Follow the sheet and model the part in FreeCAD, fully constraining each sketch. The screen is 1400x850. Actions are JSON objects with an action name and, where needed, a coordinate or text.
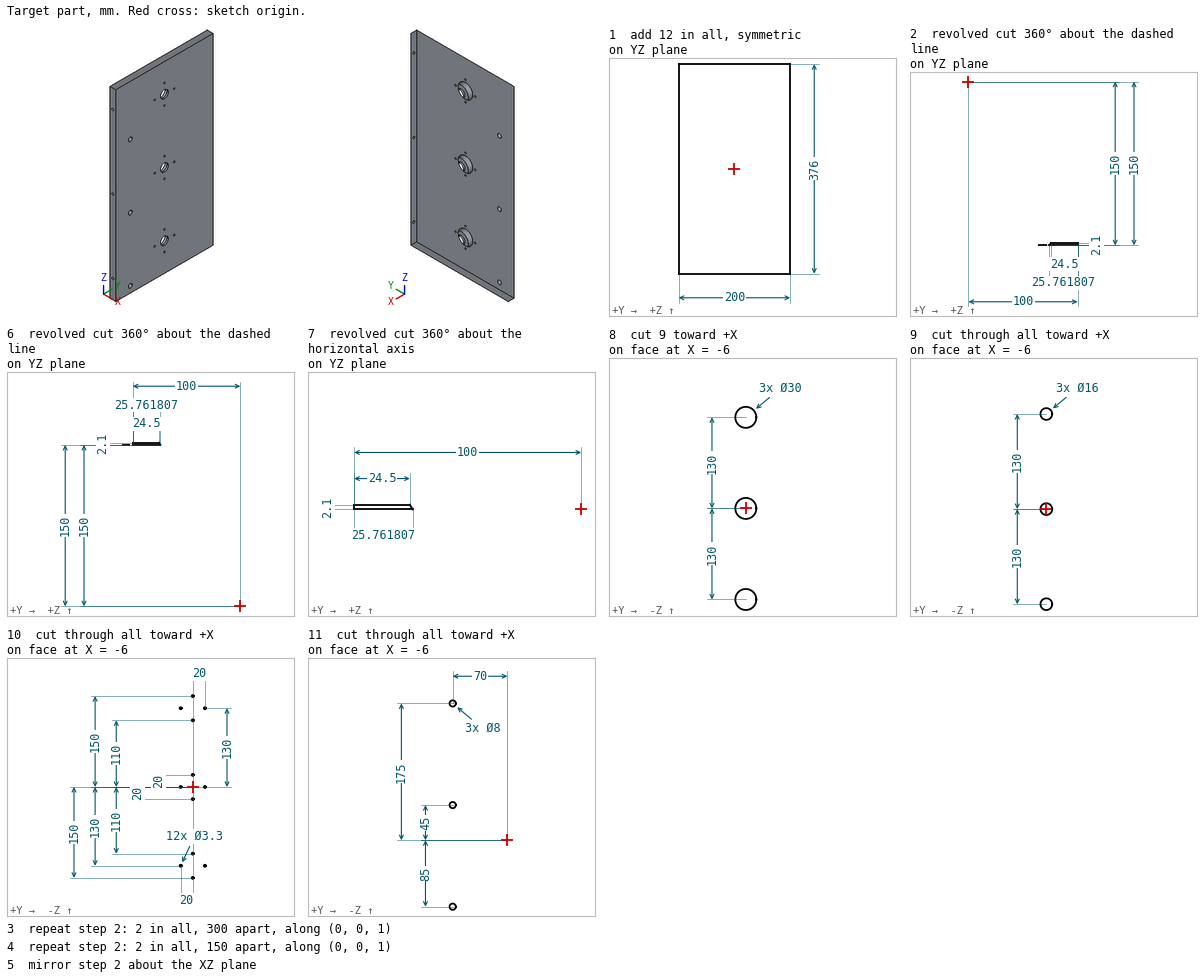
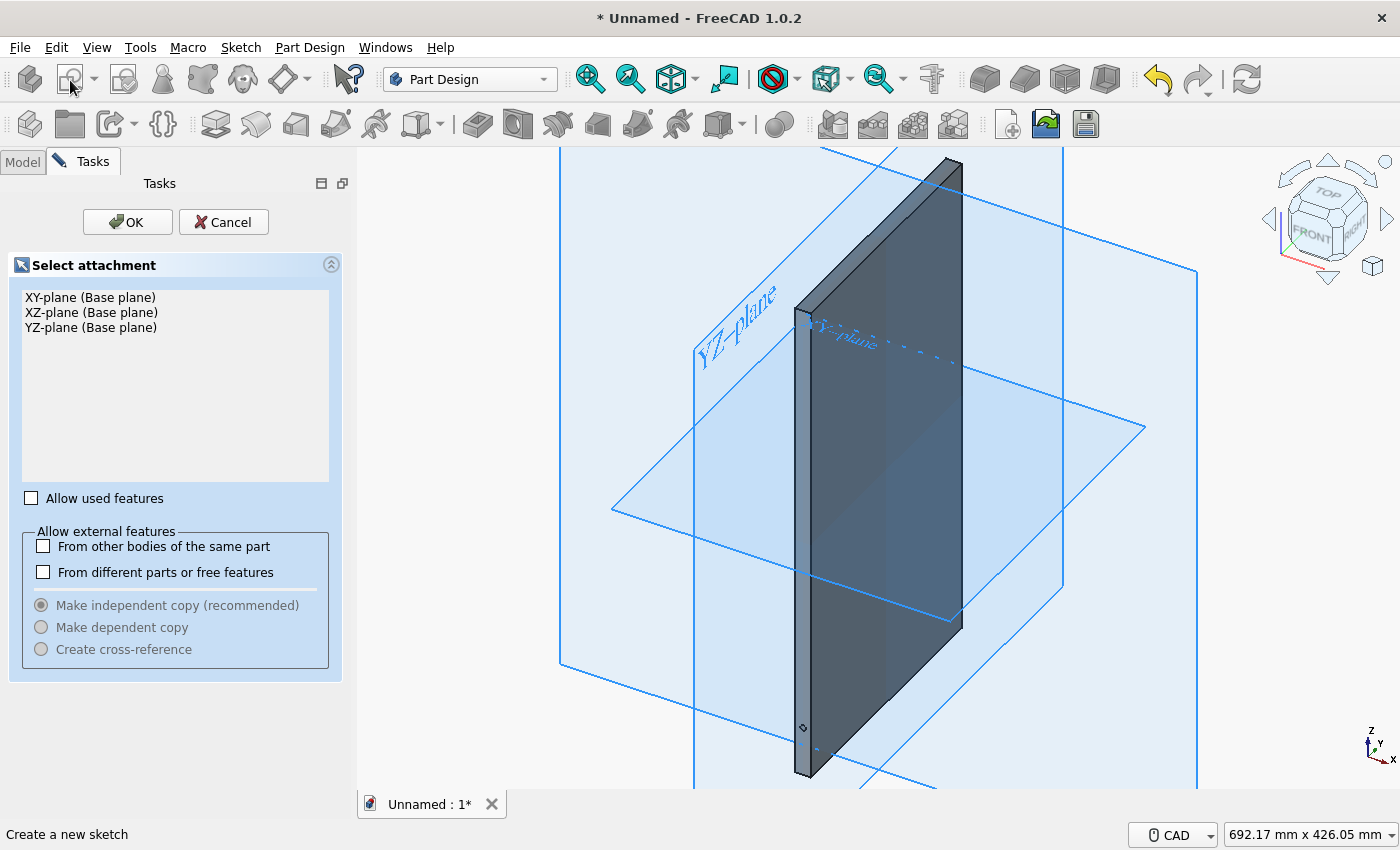
{"action": "left_click", "coordinate": [82, 328]}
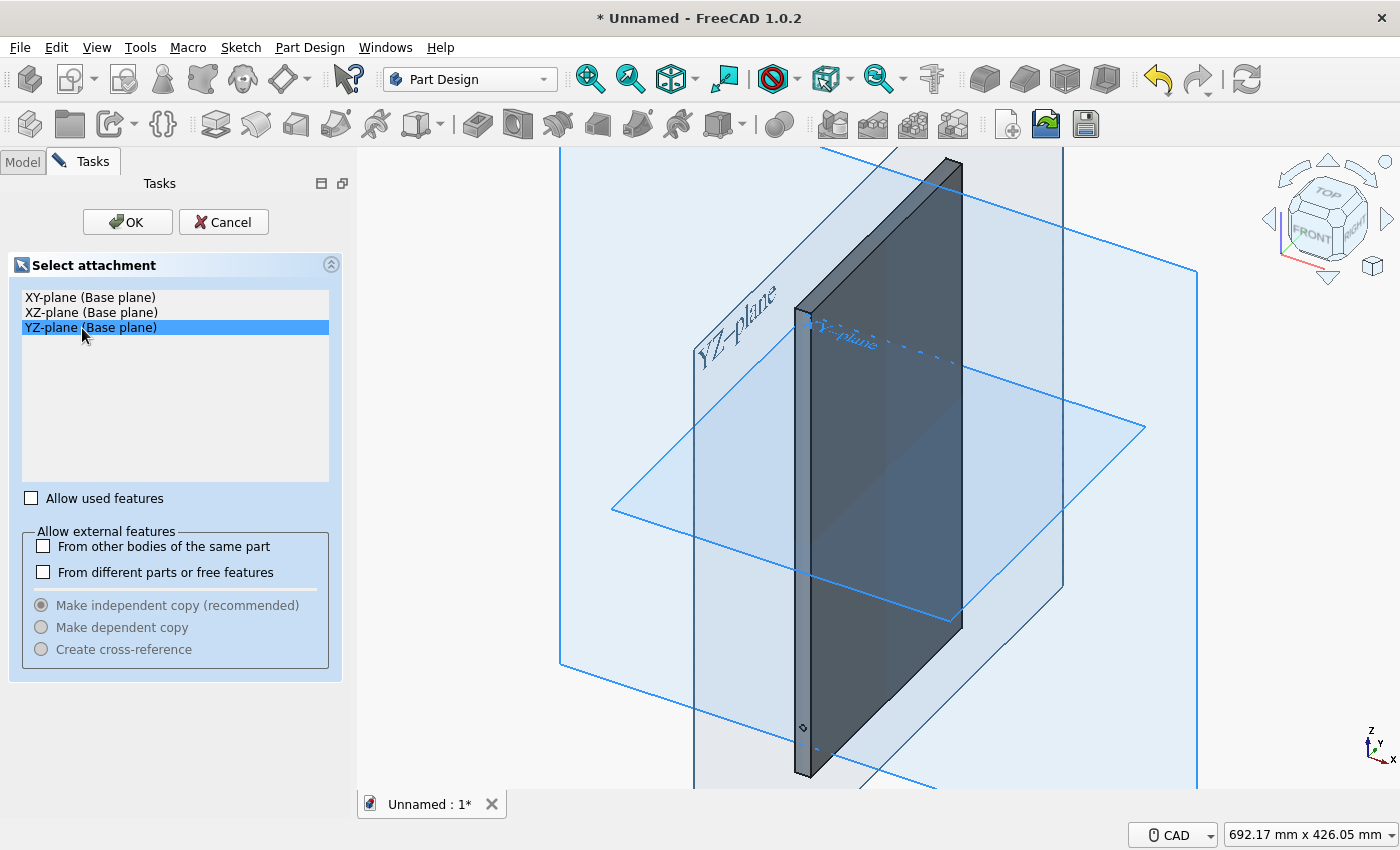
{"action": "left_click", "coordinate": [128, 222]}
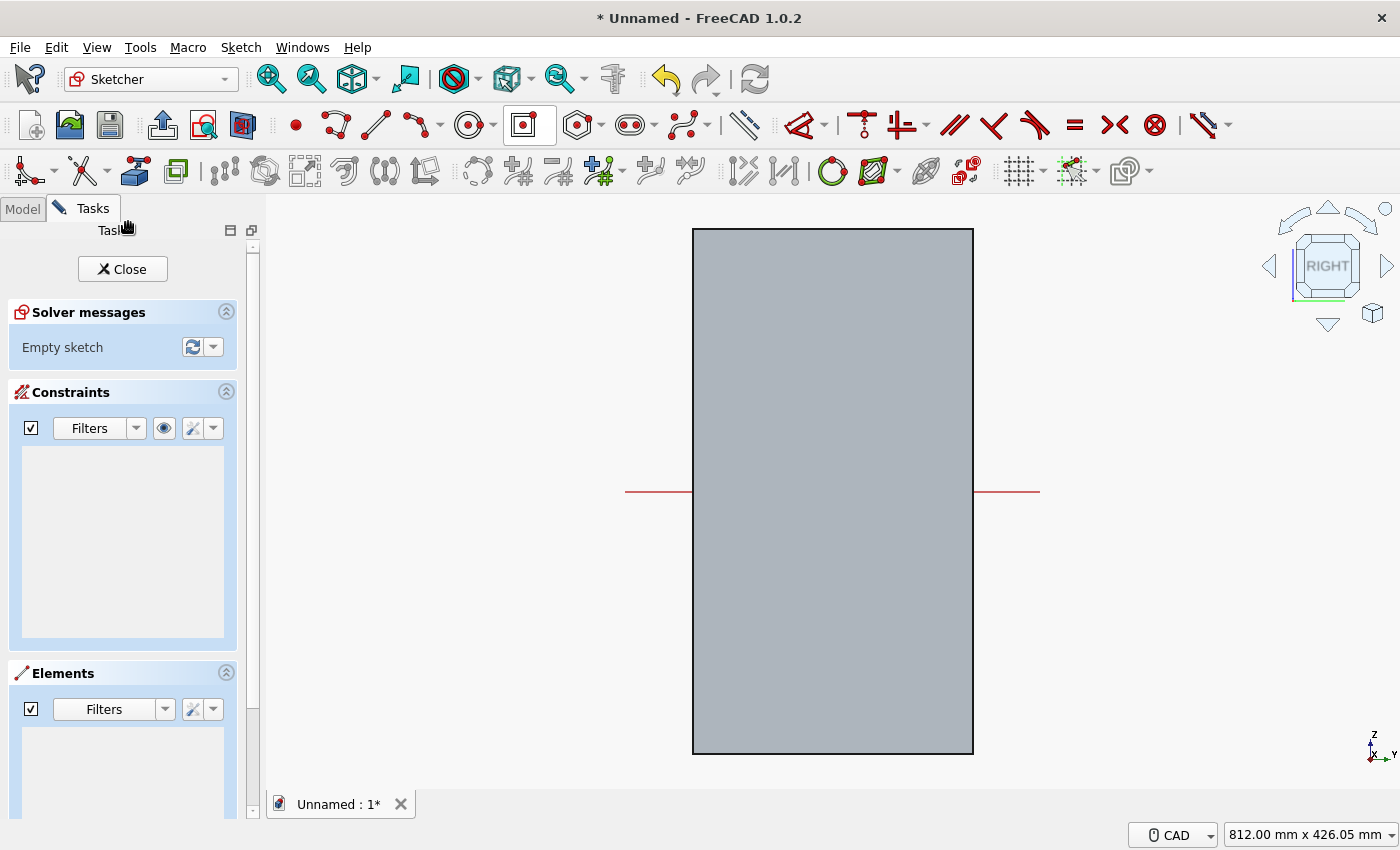
{"action": "left_click", "coordinate": [244, 126]}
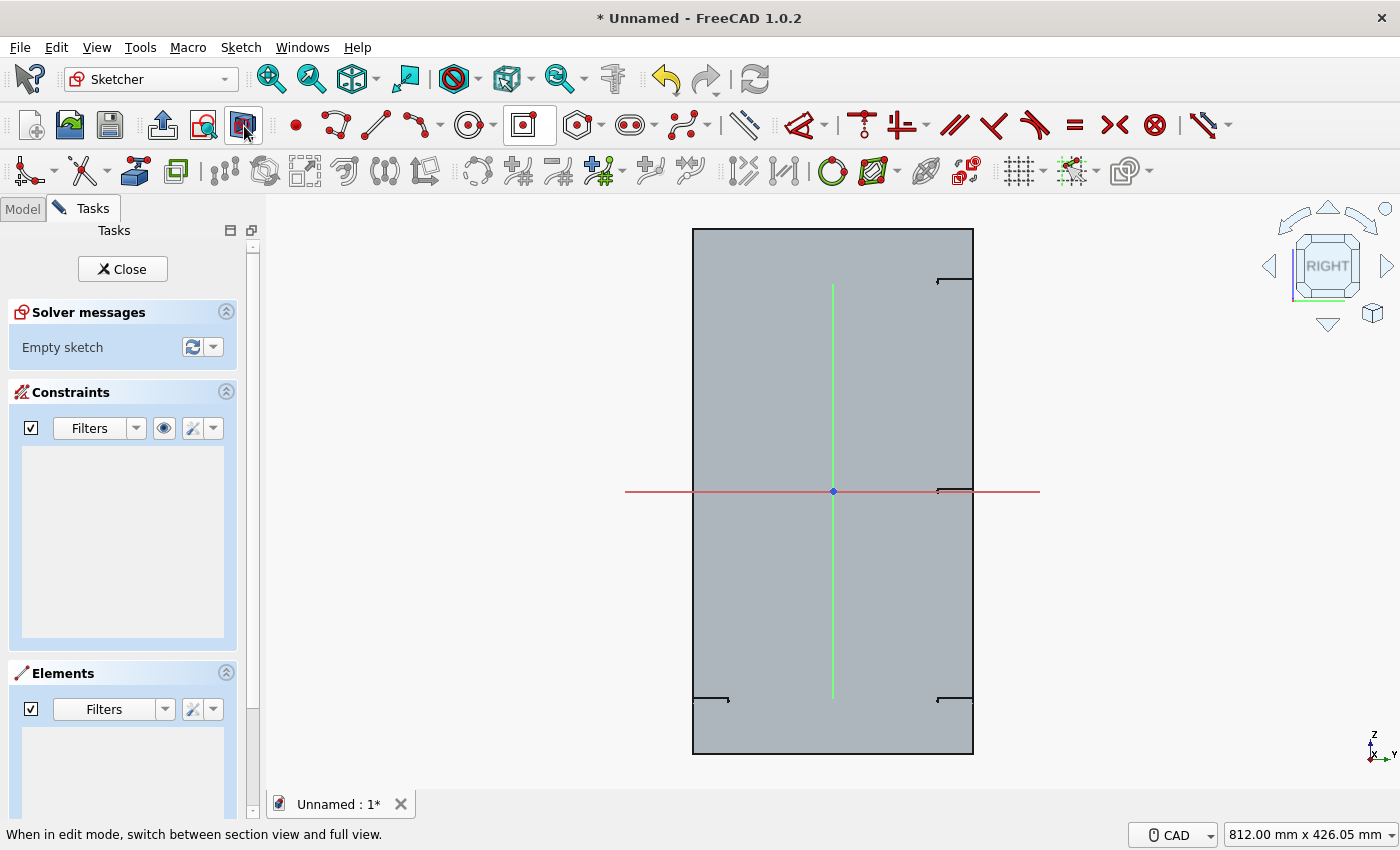
{"action": "scroll", "coordinate": [699, 264], "scroll_direction": "up", "scroll_amount": 13}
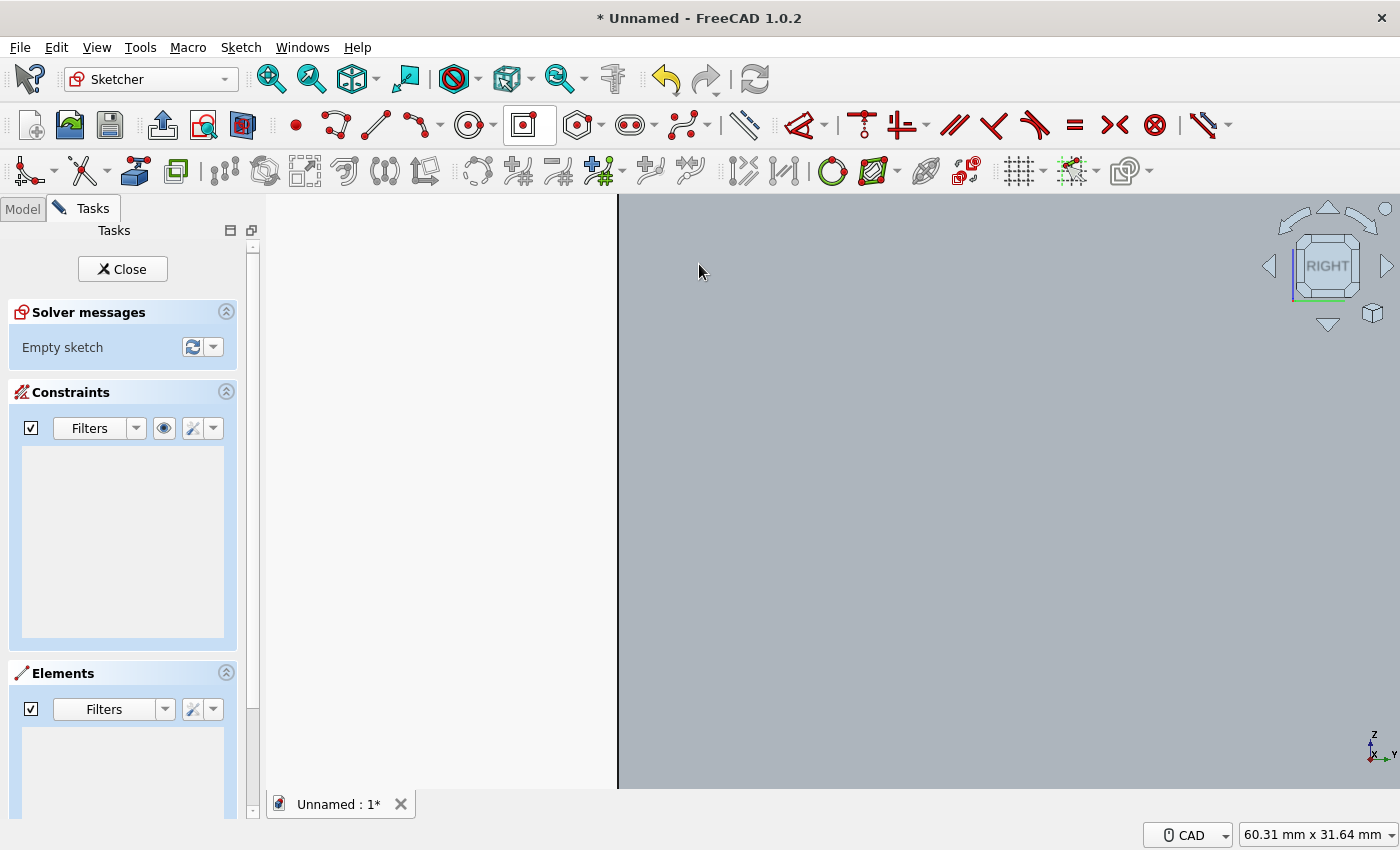
{"action": "left_click", "coordinate": [336, 126]}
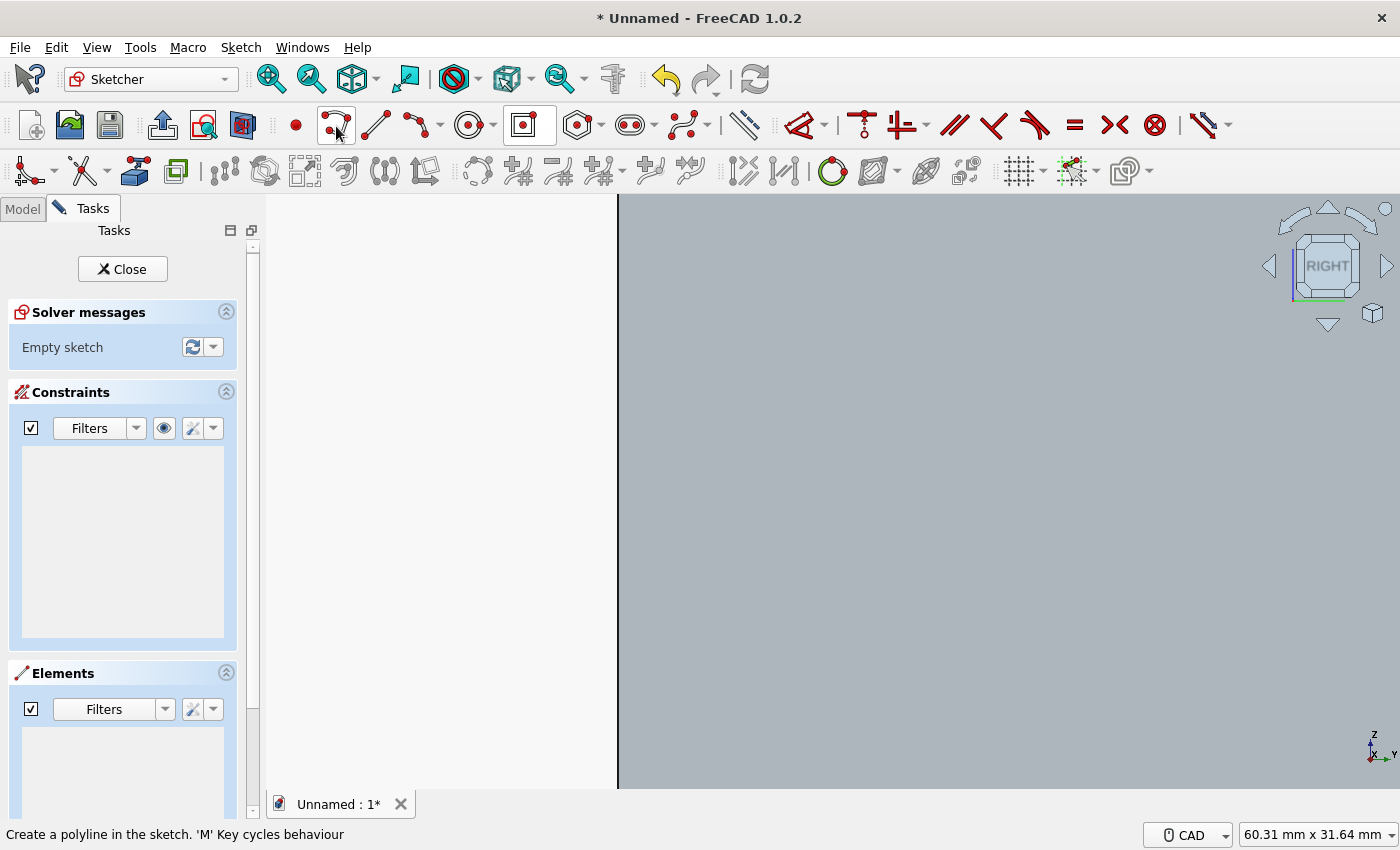
{"action": "left_click", "coordinate": [1102, 505]}
{"action": "left_click", "coordinate": [1079, 466]}
{"action": "left_click", "coordinate": [618, 466]}
{"action": "left_click", "coordinate": [618, 505]}
{"action": "left_click", "coordinate": [1102, 506]}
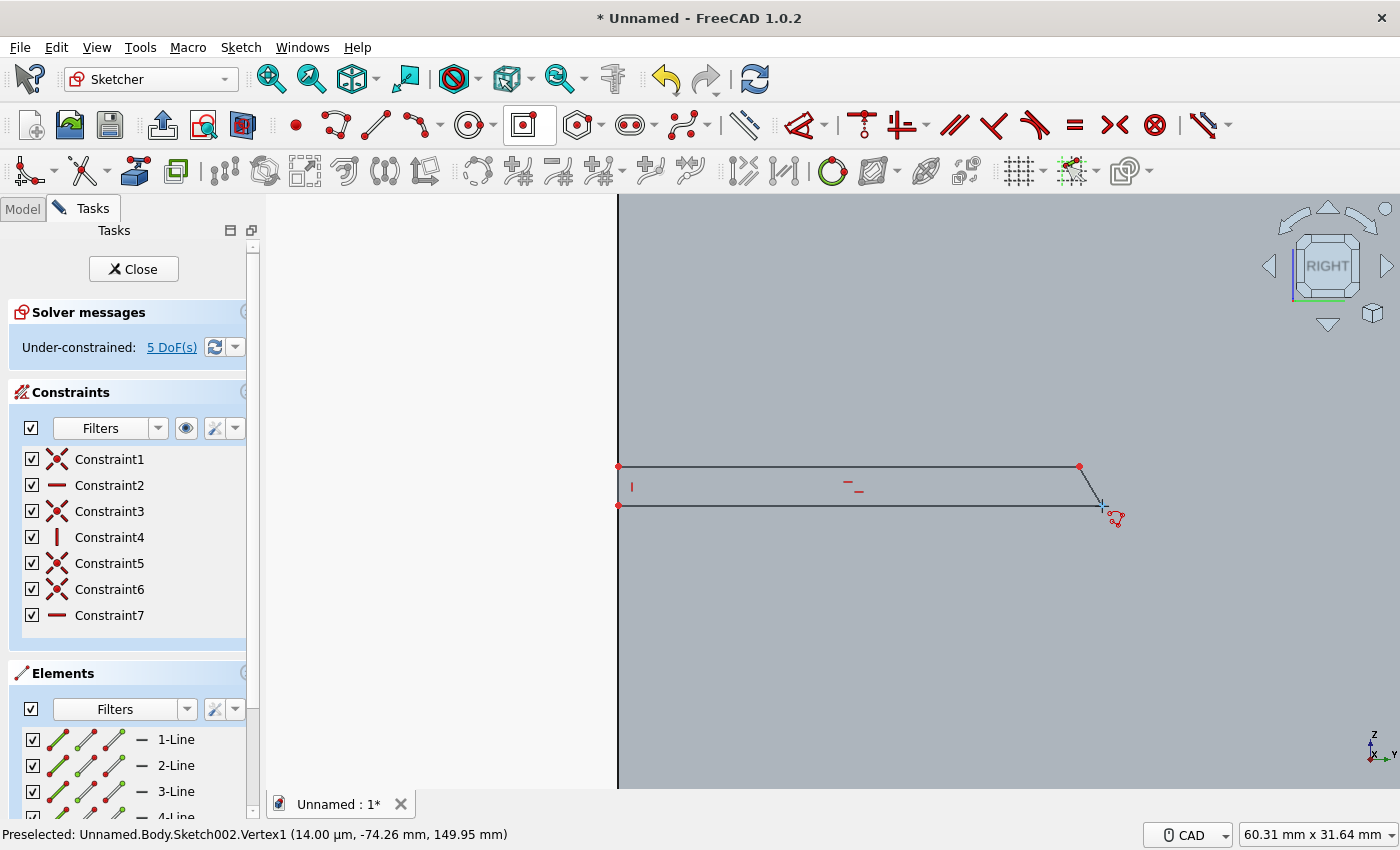
{"action": "left_click", "coordinate": [376, 126]}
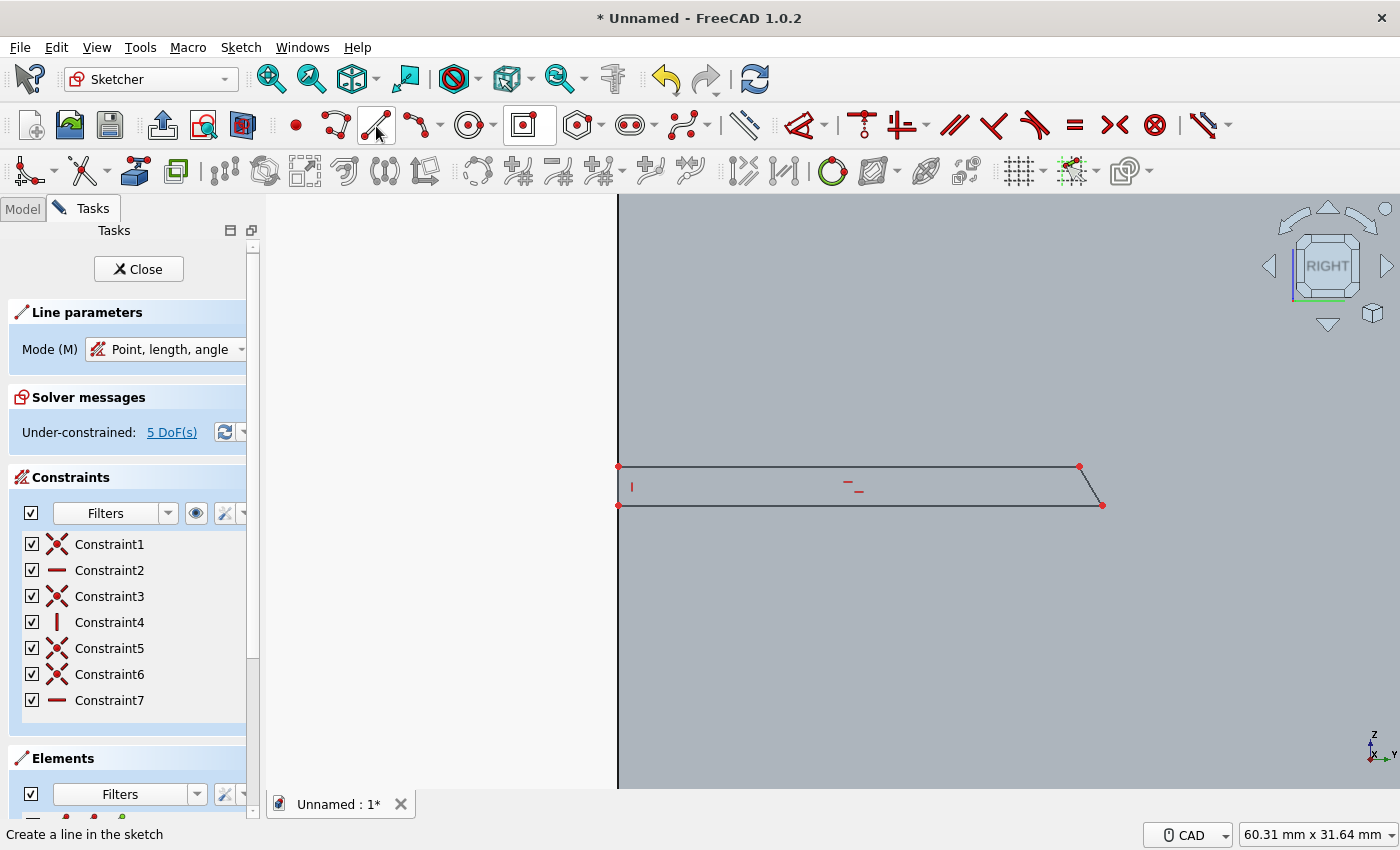
{"action": "left_click", "coordinate": [570, 505]}
{"action": "left_click", "coordinate": [424, 505]}
{"action": "key", "text": "Escape"}